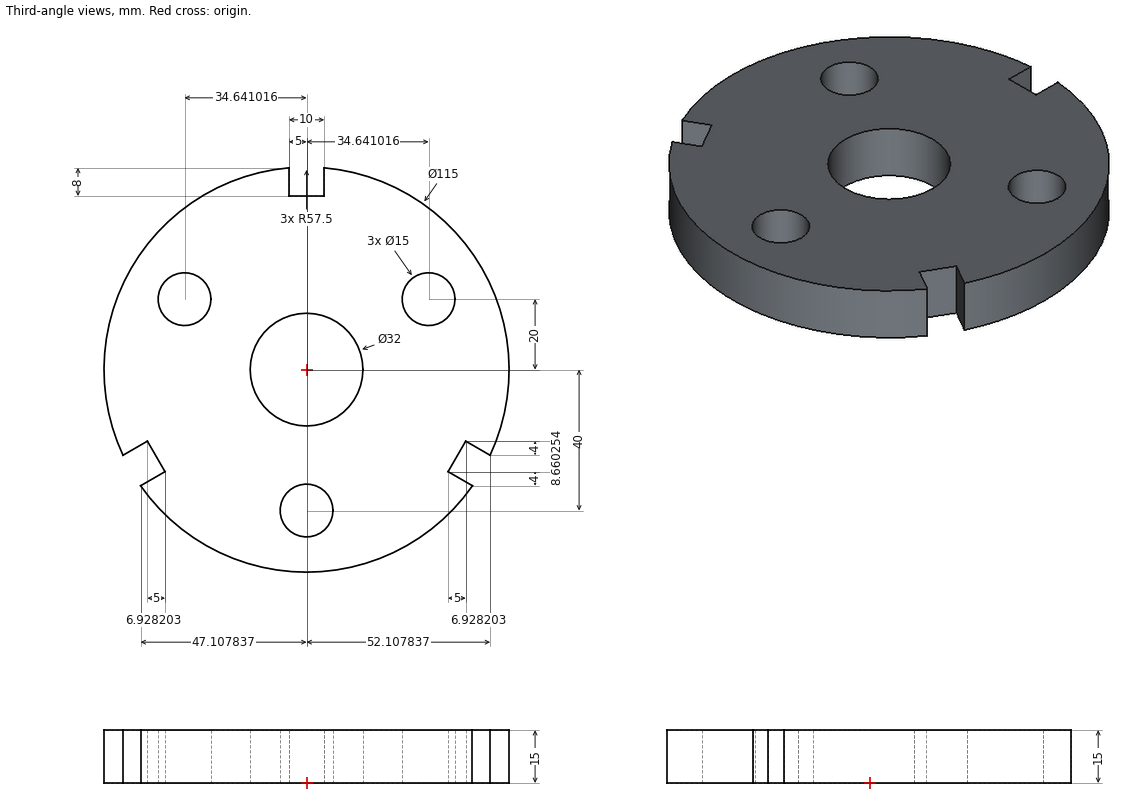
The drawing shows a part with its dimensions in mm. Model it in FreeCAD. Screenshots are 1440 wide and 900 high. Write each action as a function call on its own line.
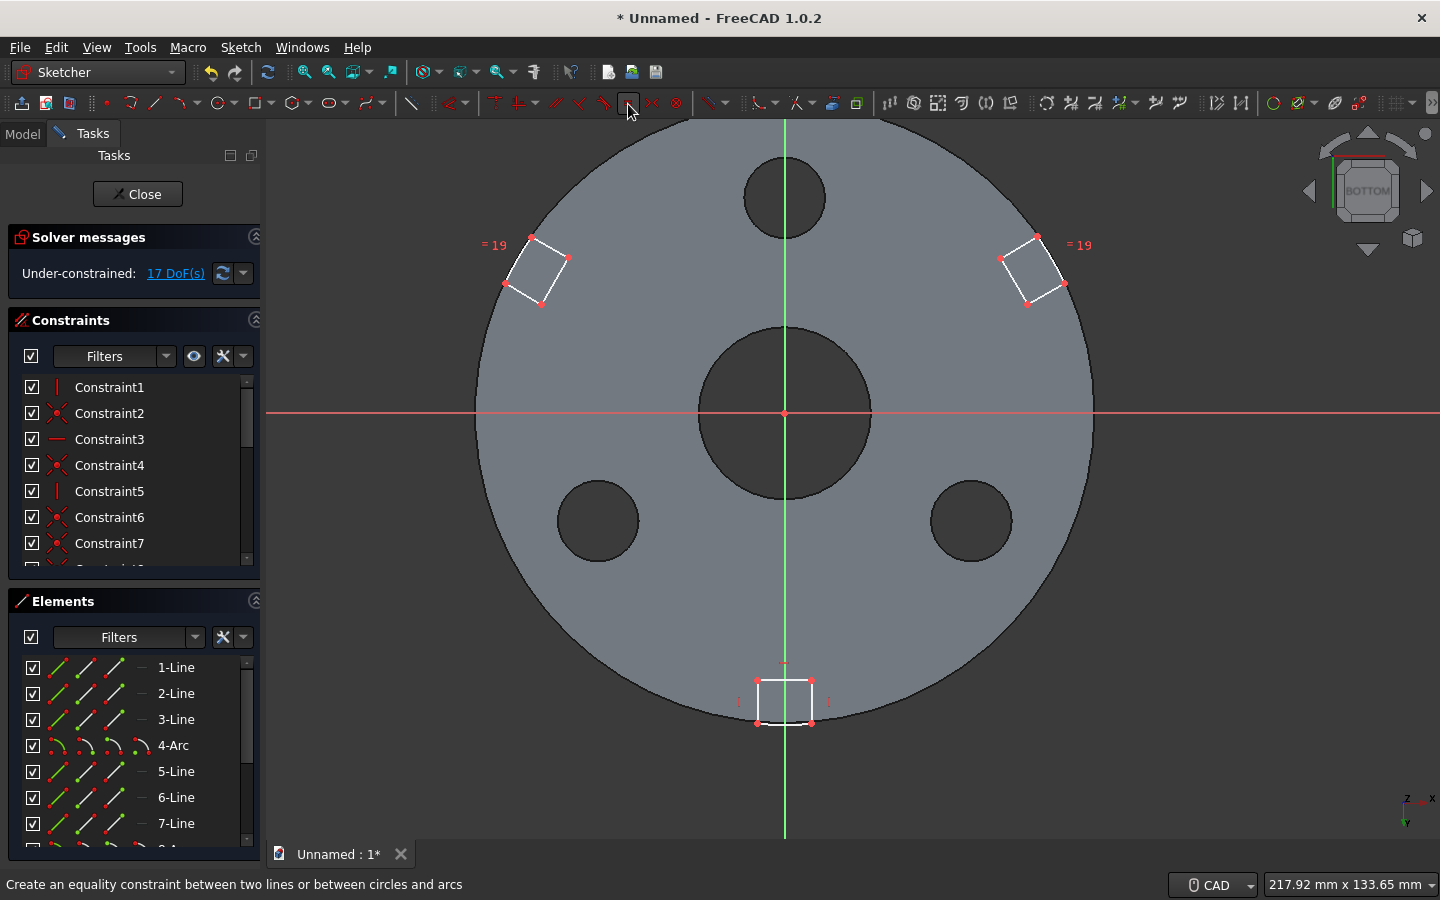
click(450, 104)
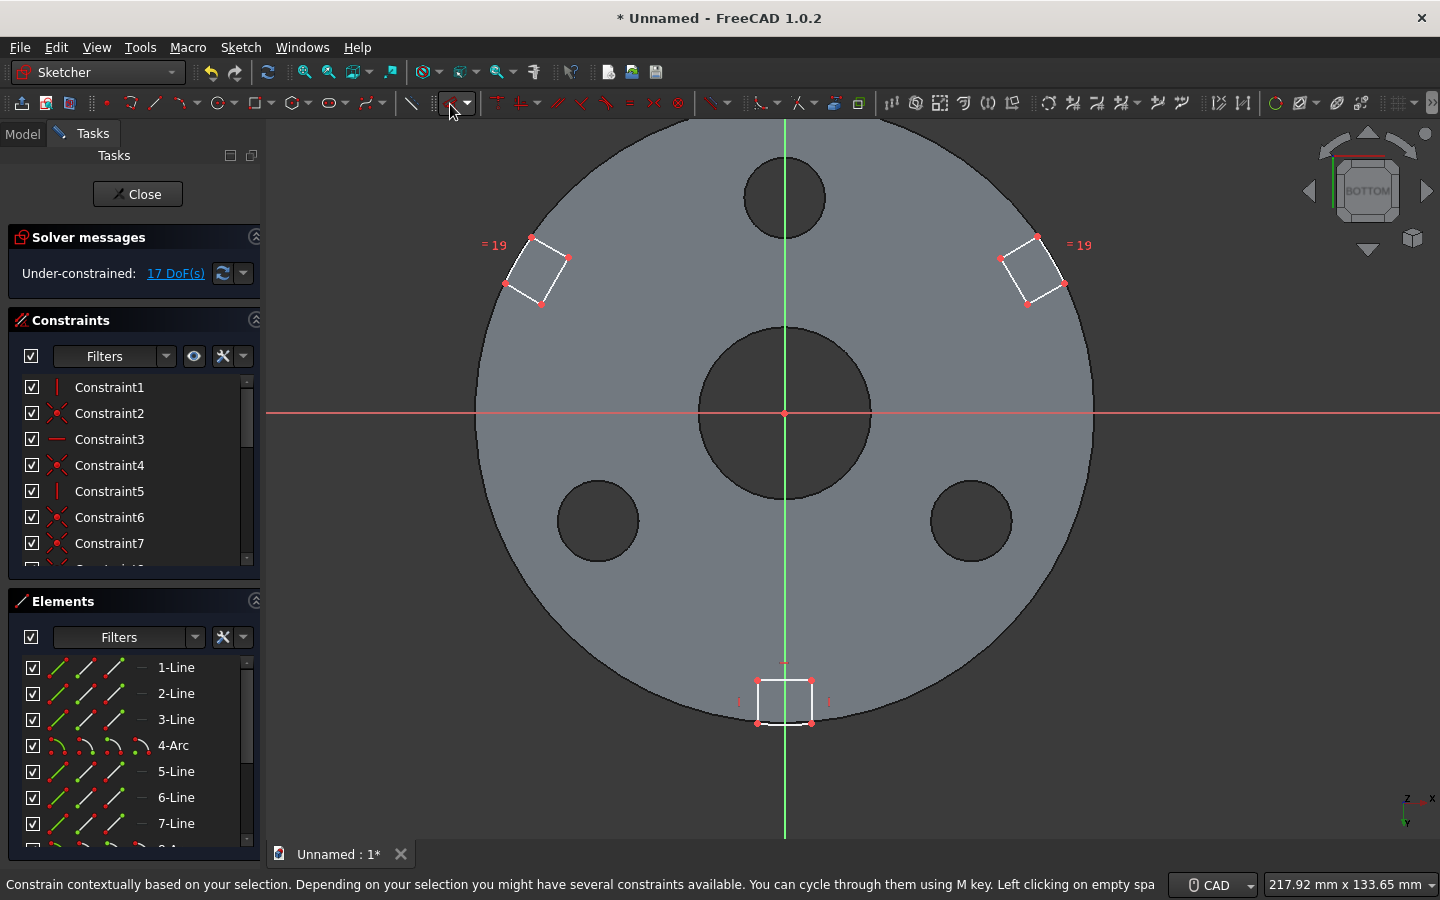
scroll(774, 725, up, 2)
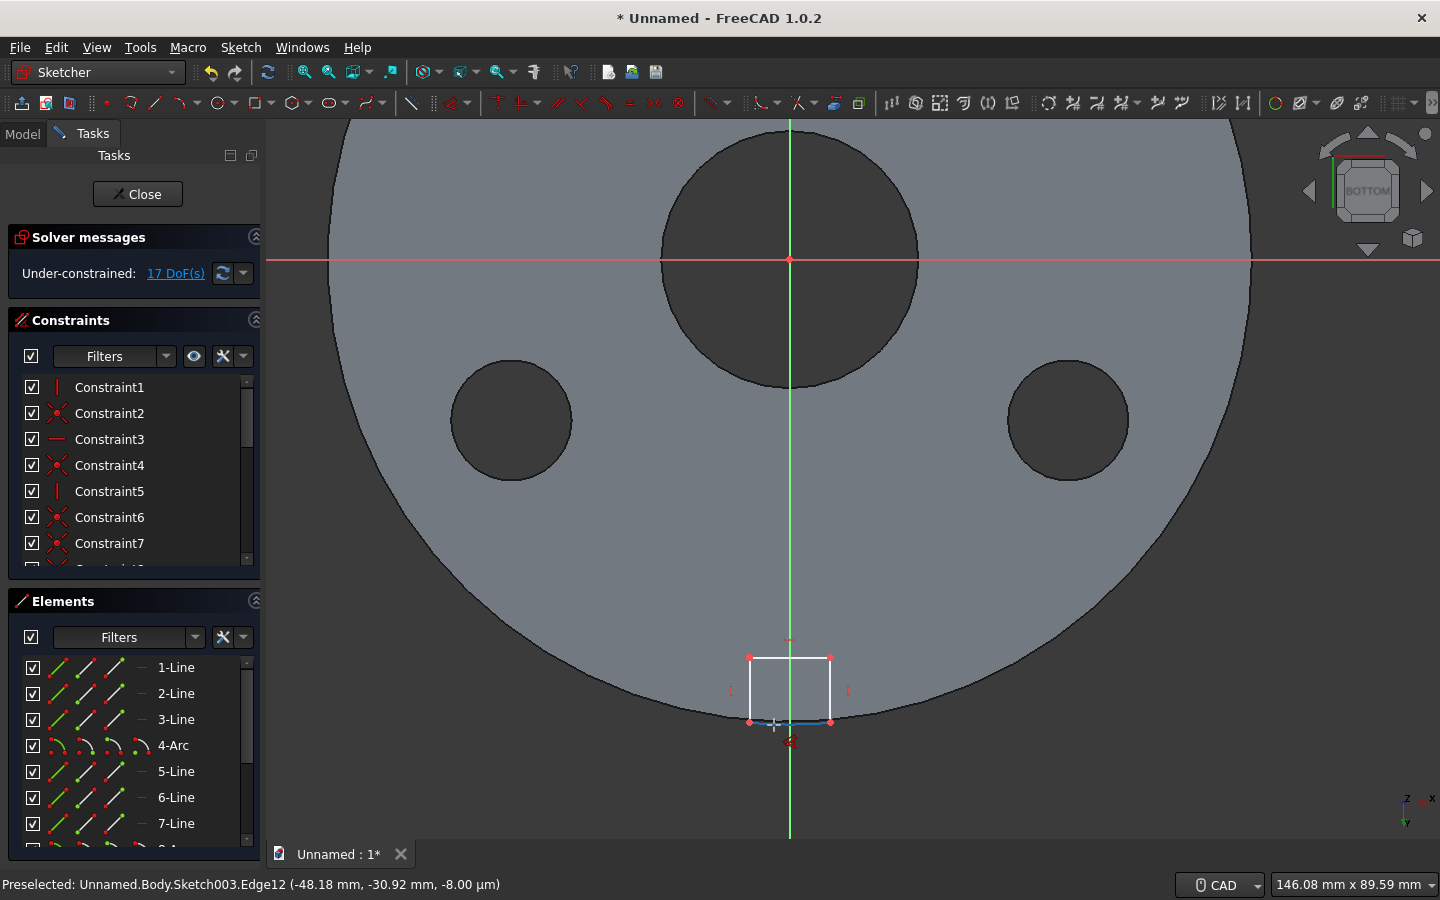
click(774, 724)
click(773, 756)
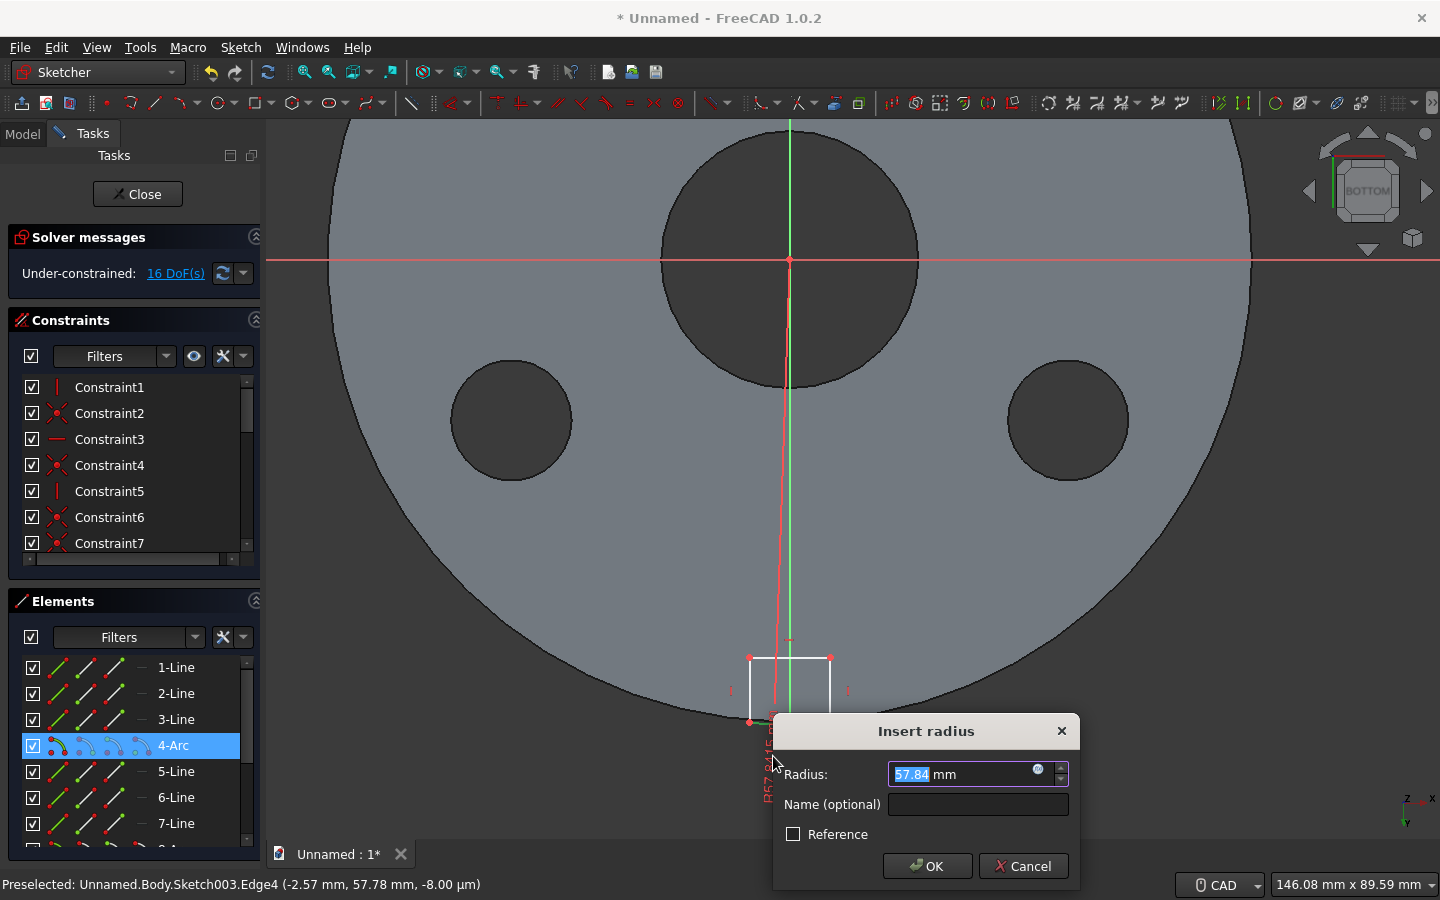
text(57.5)
key(Return)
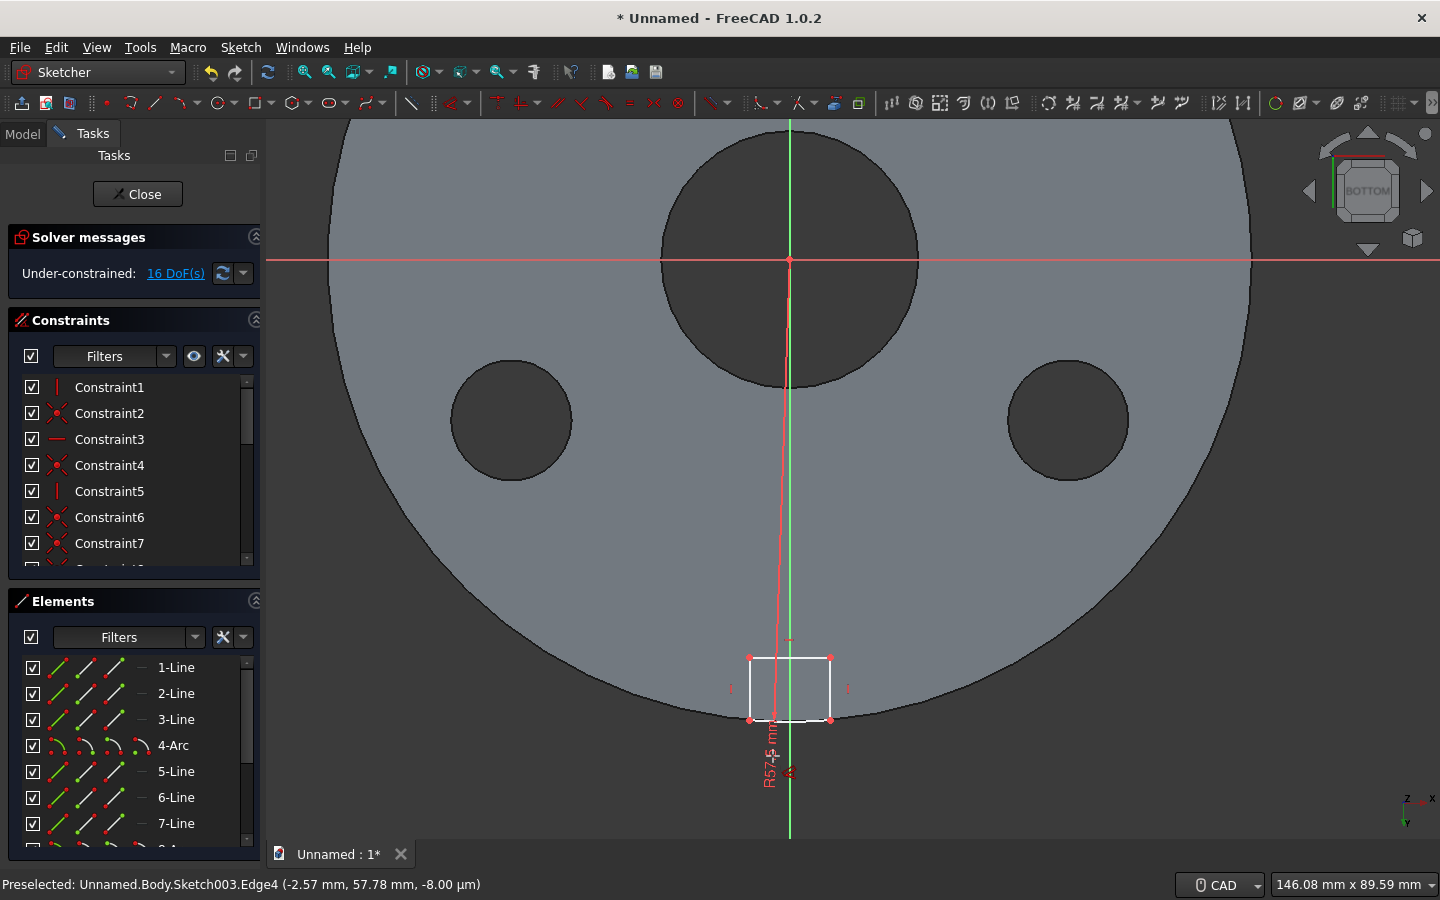
scroll(774, 725, down, 2)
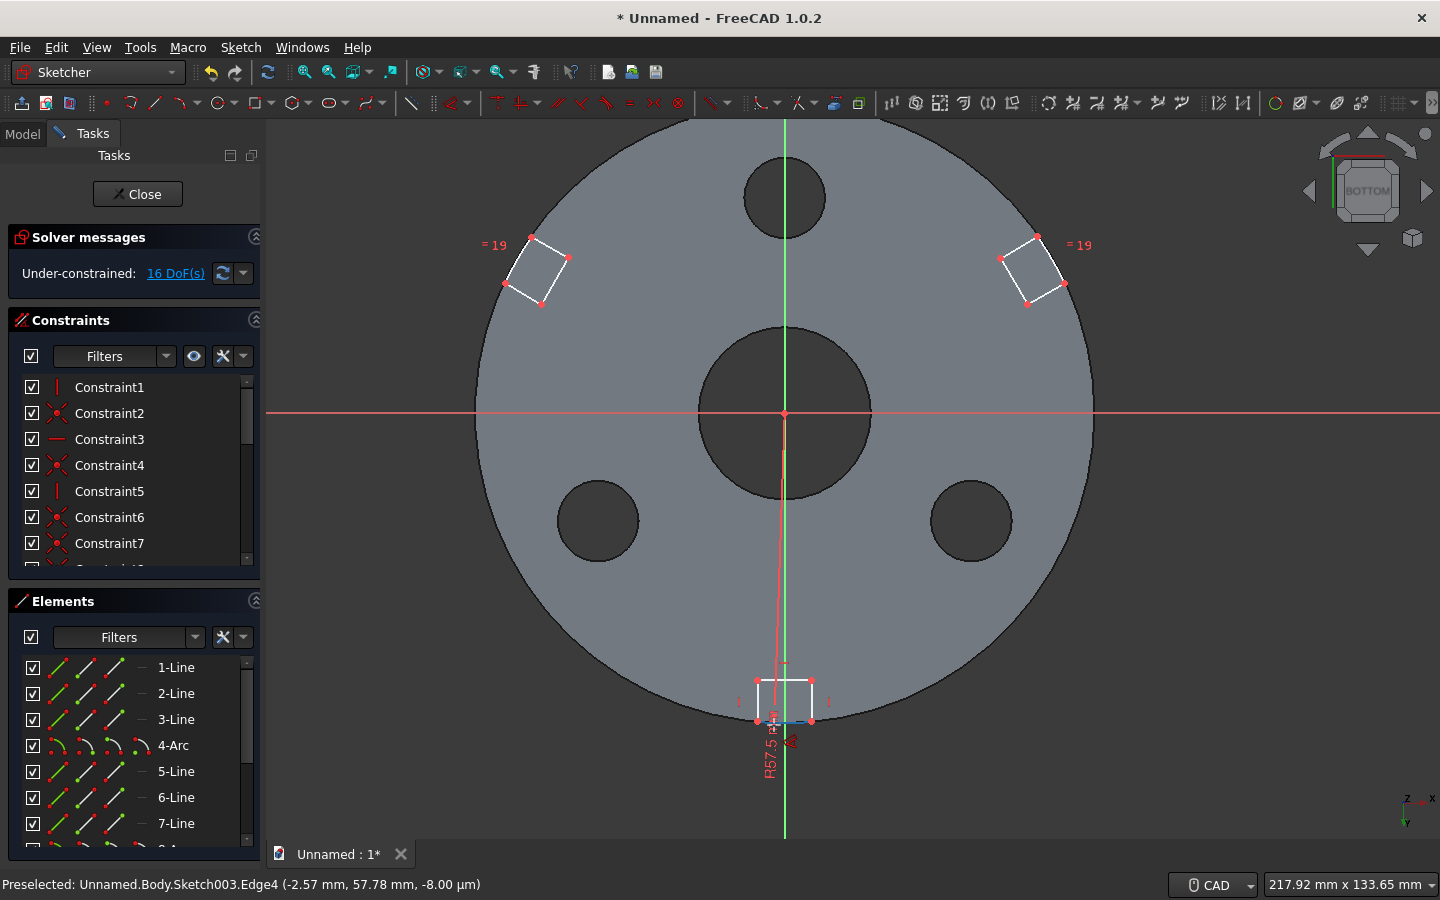
click(1057, 269)
click(1085, 254)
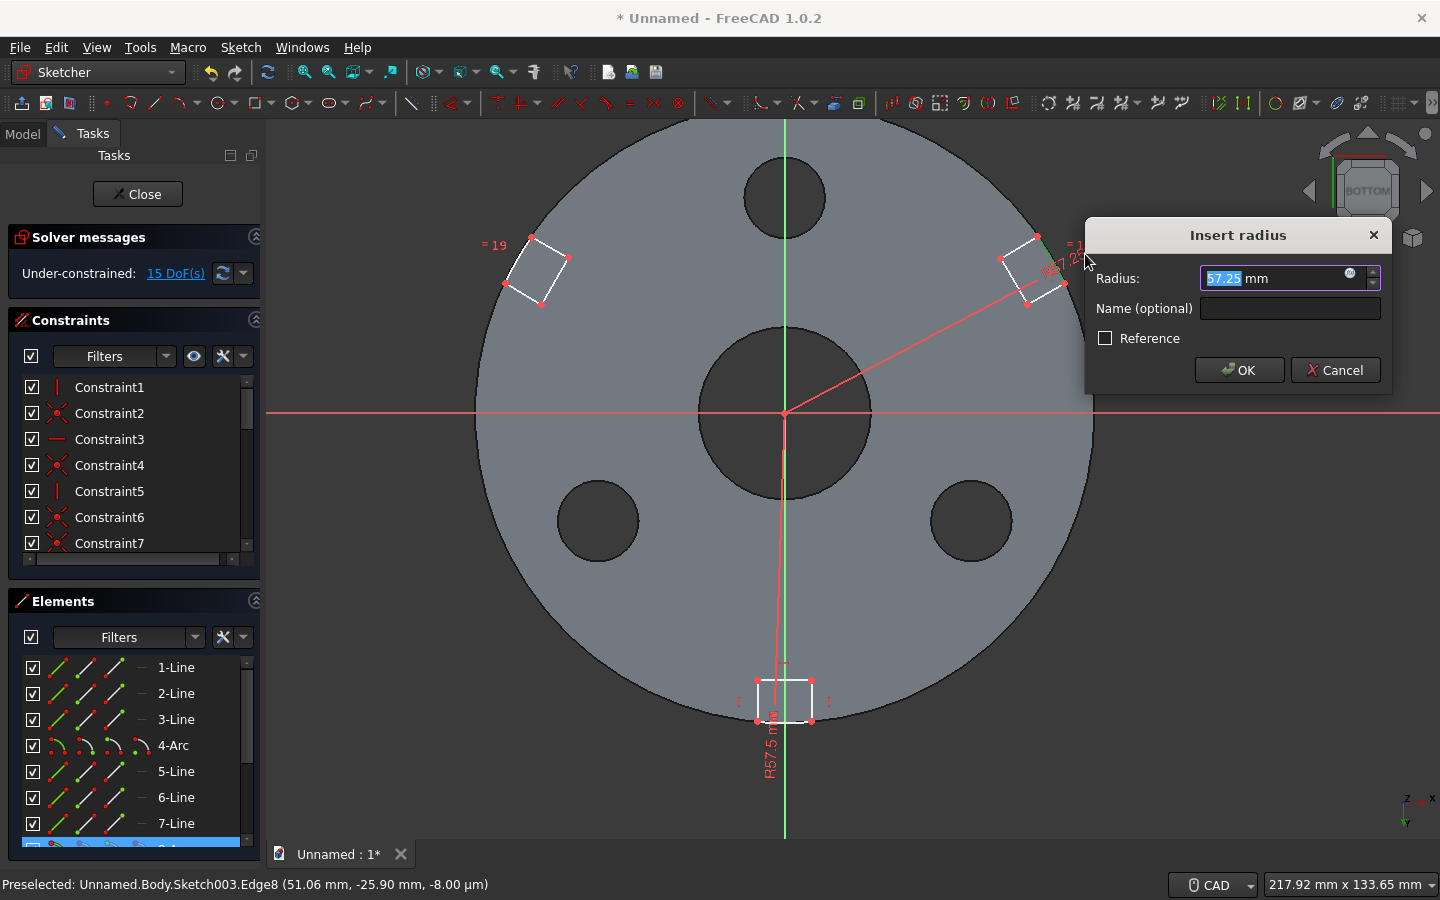
text(57.5)
key(Return)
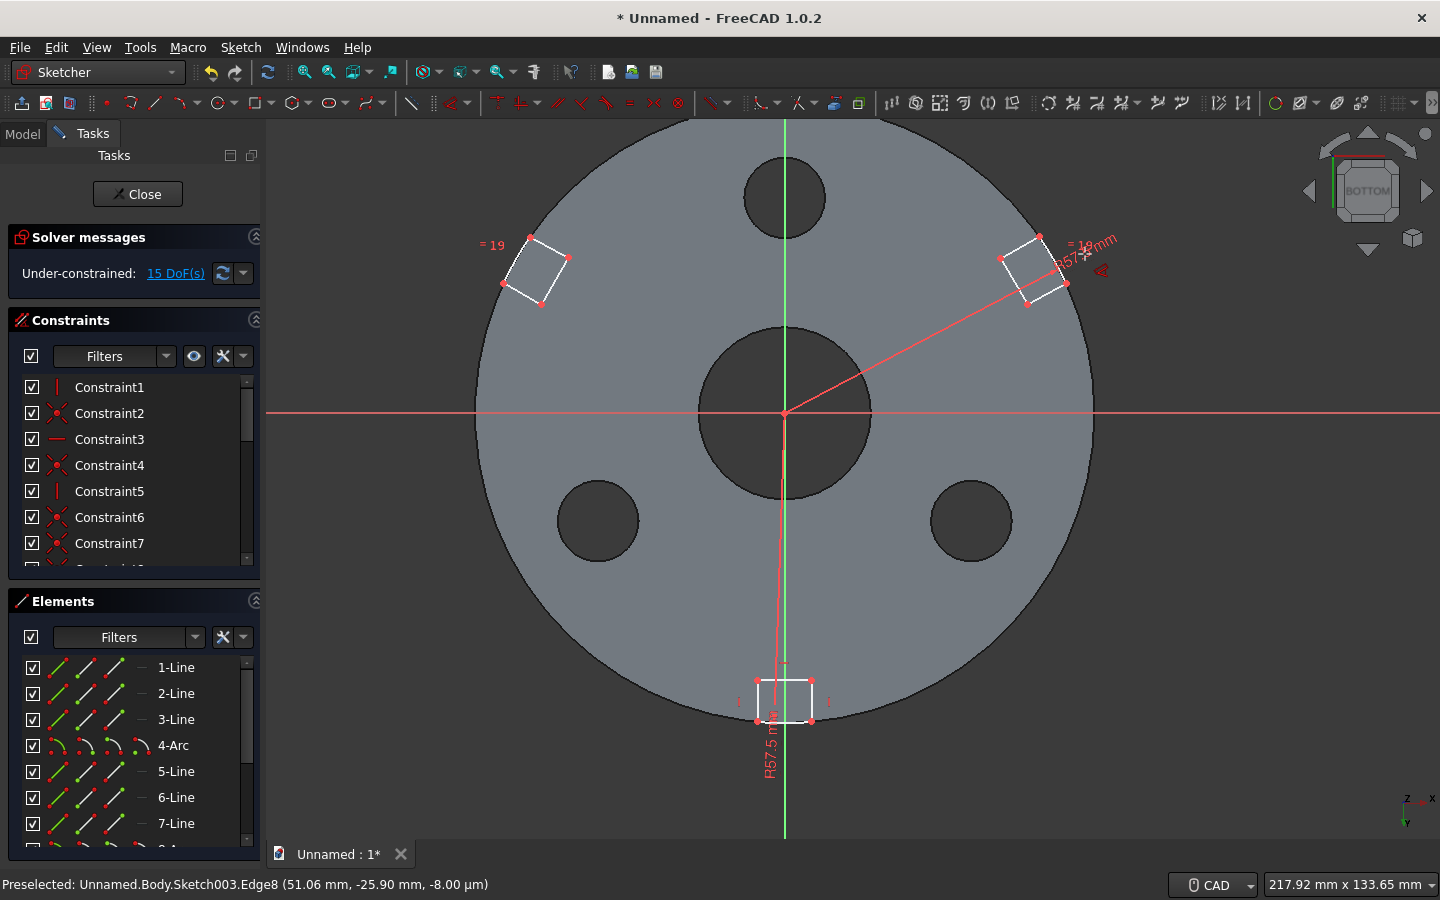
click(758, 709)
click(724, 701)